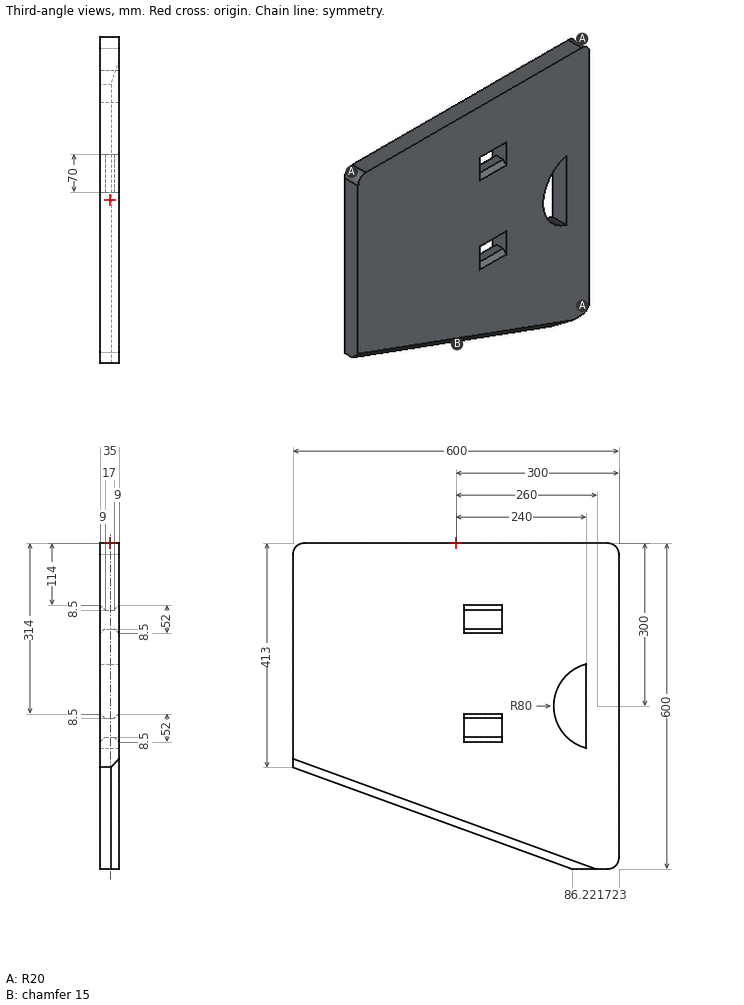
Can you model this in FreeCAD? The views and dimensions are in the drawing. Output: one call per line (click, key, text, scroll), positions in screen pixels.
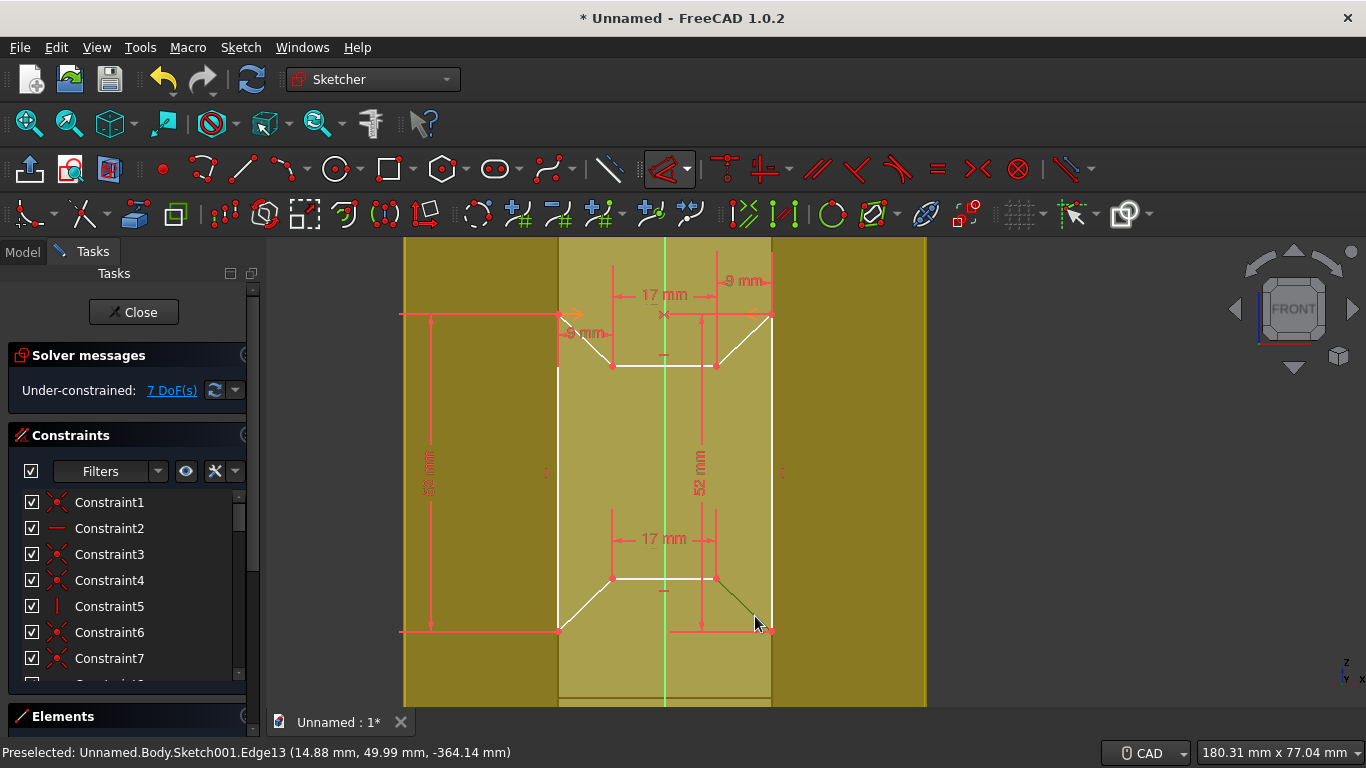
click(690, 170)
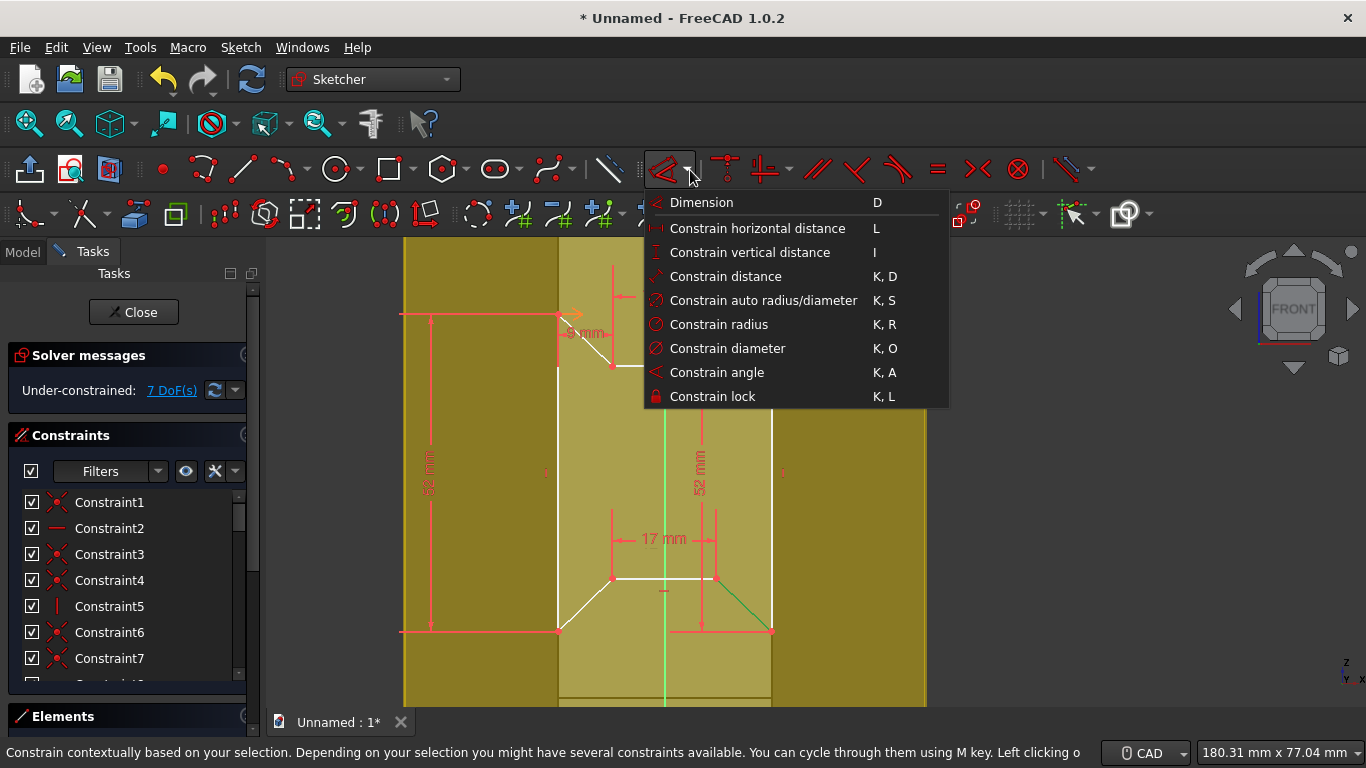
click(797, 228)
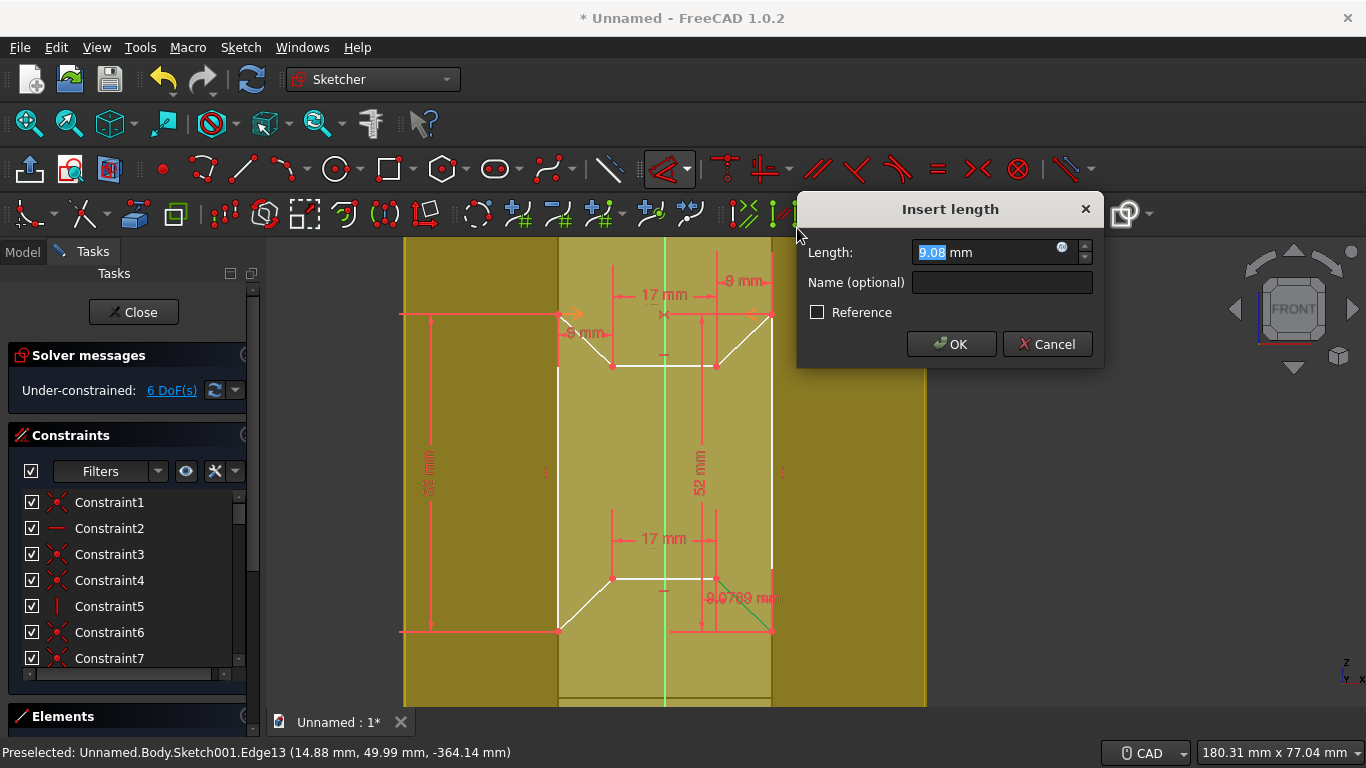
text(9)
key(Return)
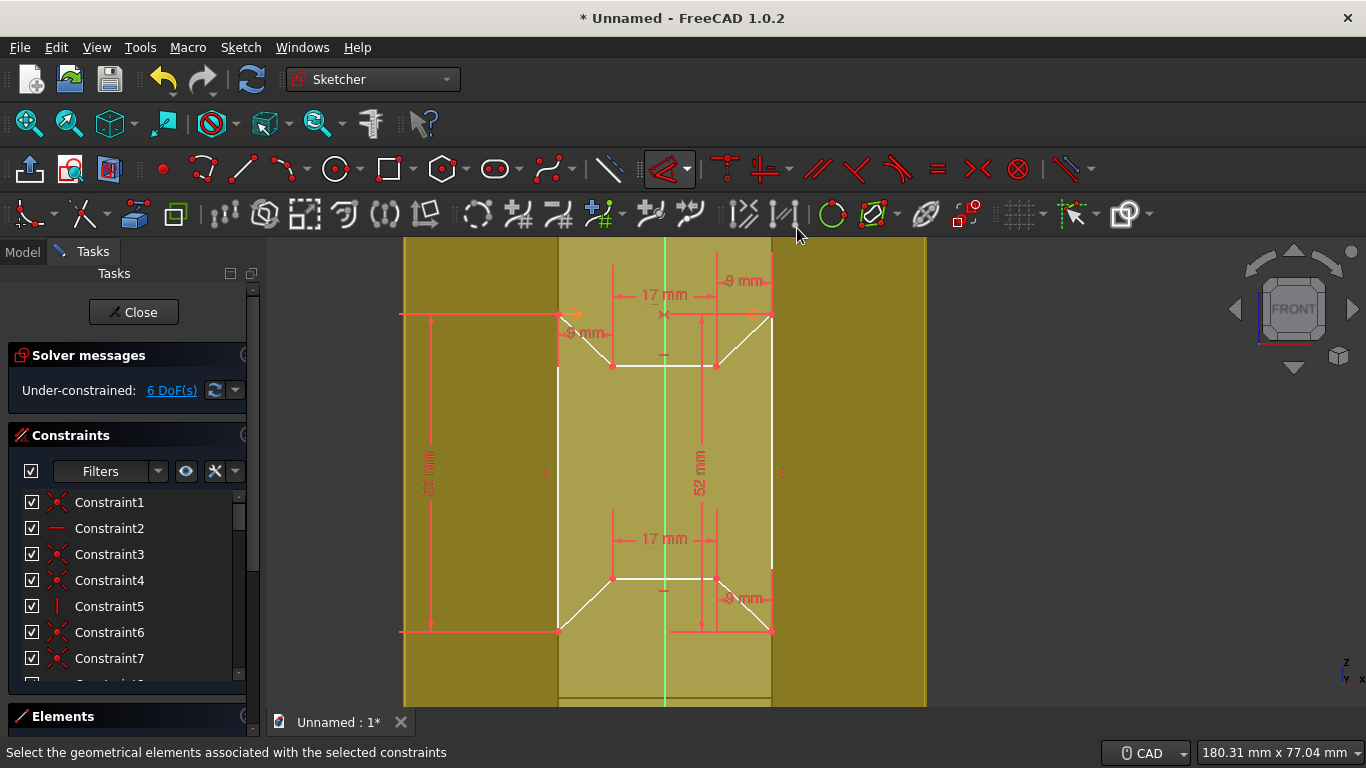
scroll(760, 622, down, 10)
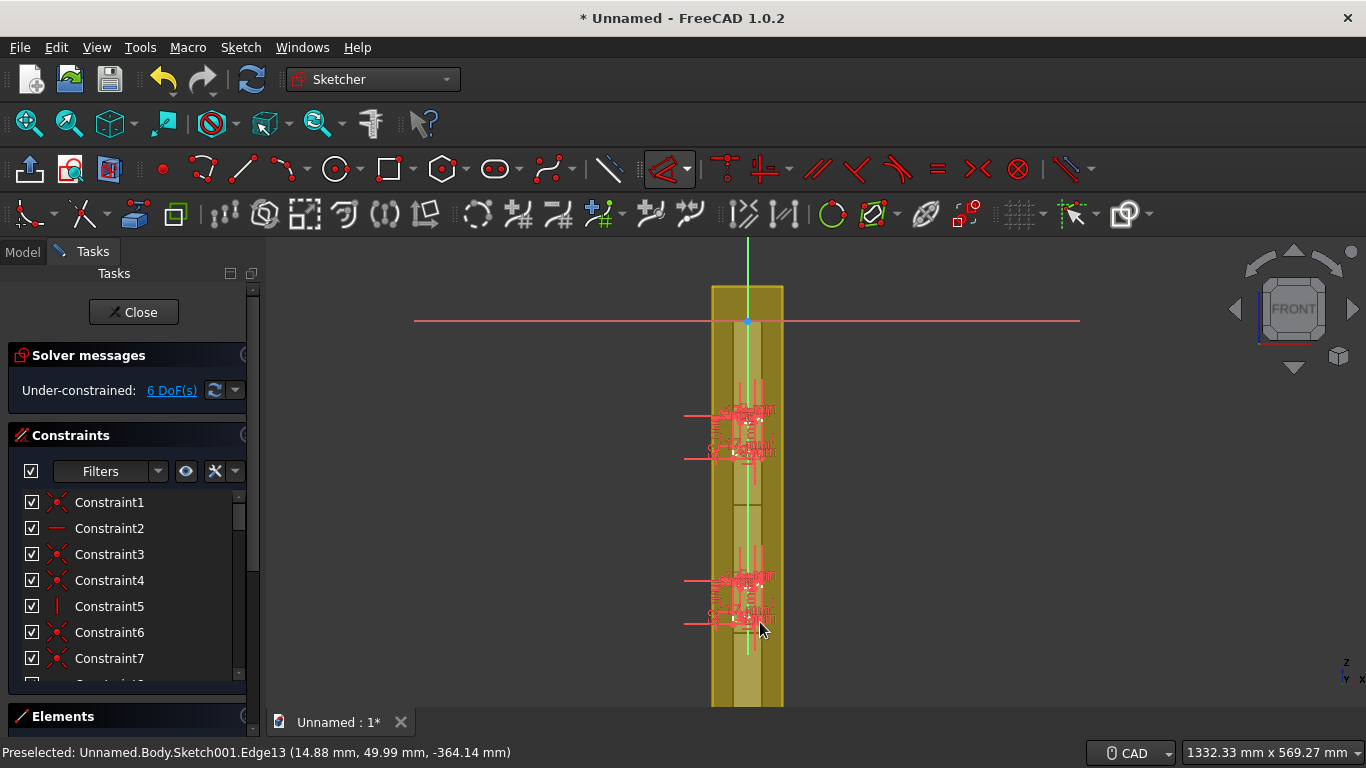
click(733, 416)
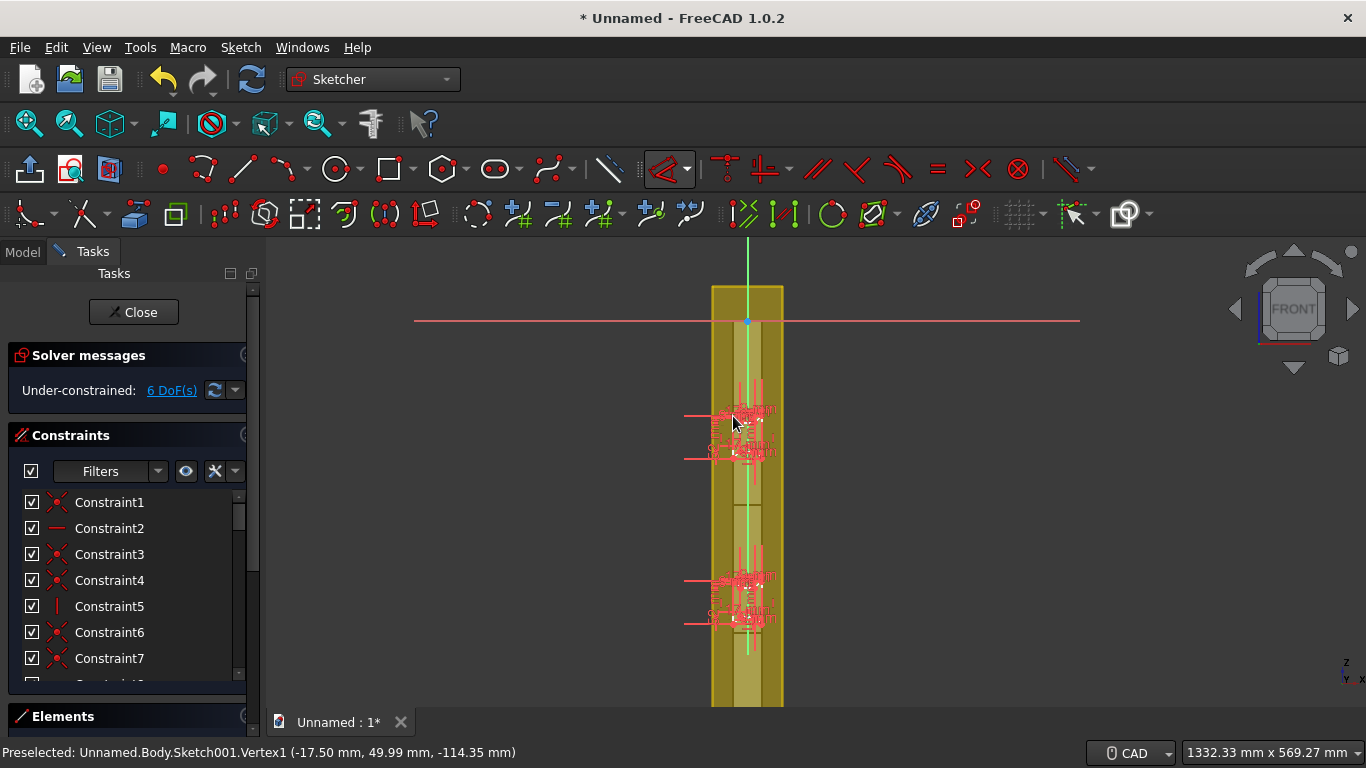
click(690, 170)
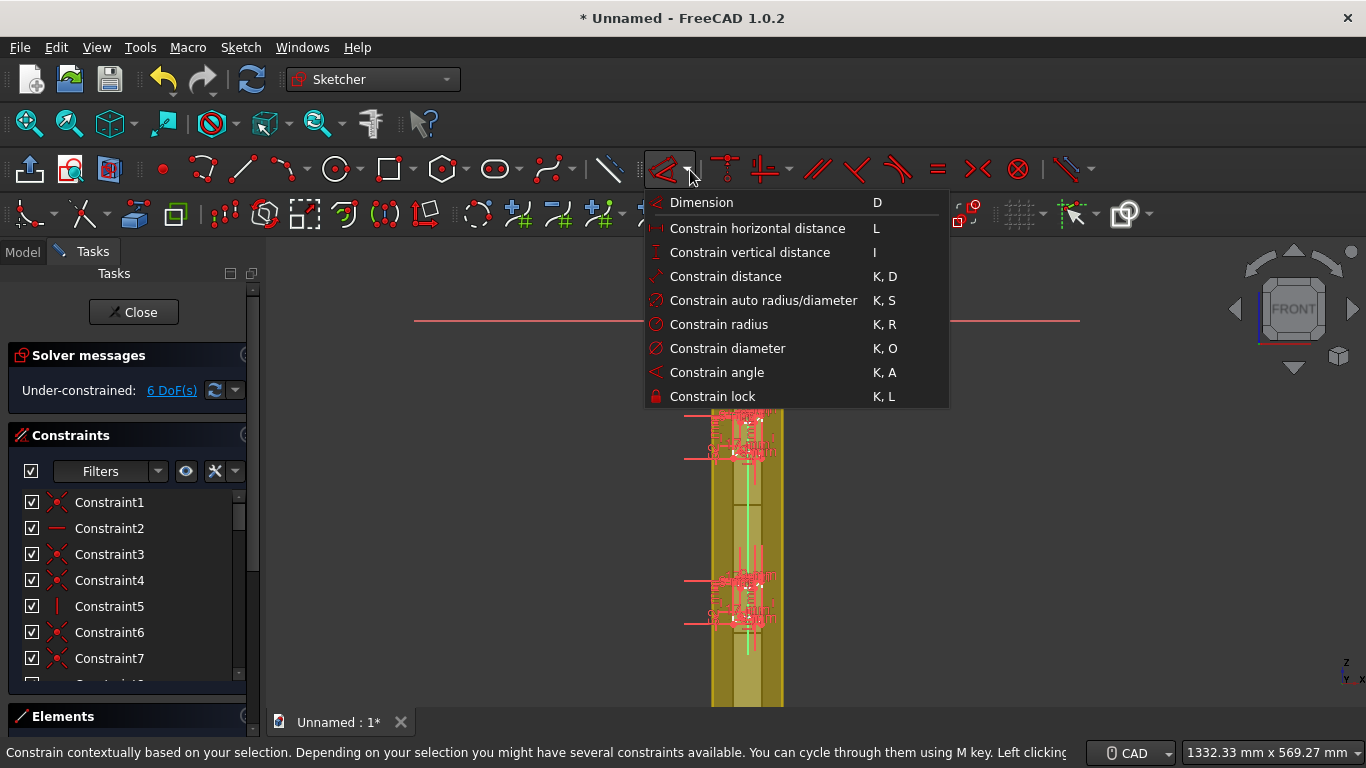
click(797, 252)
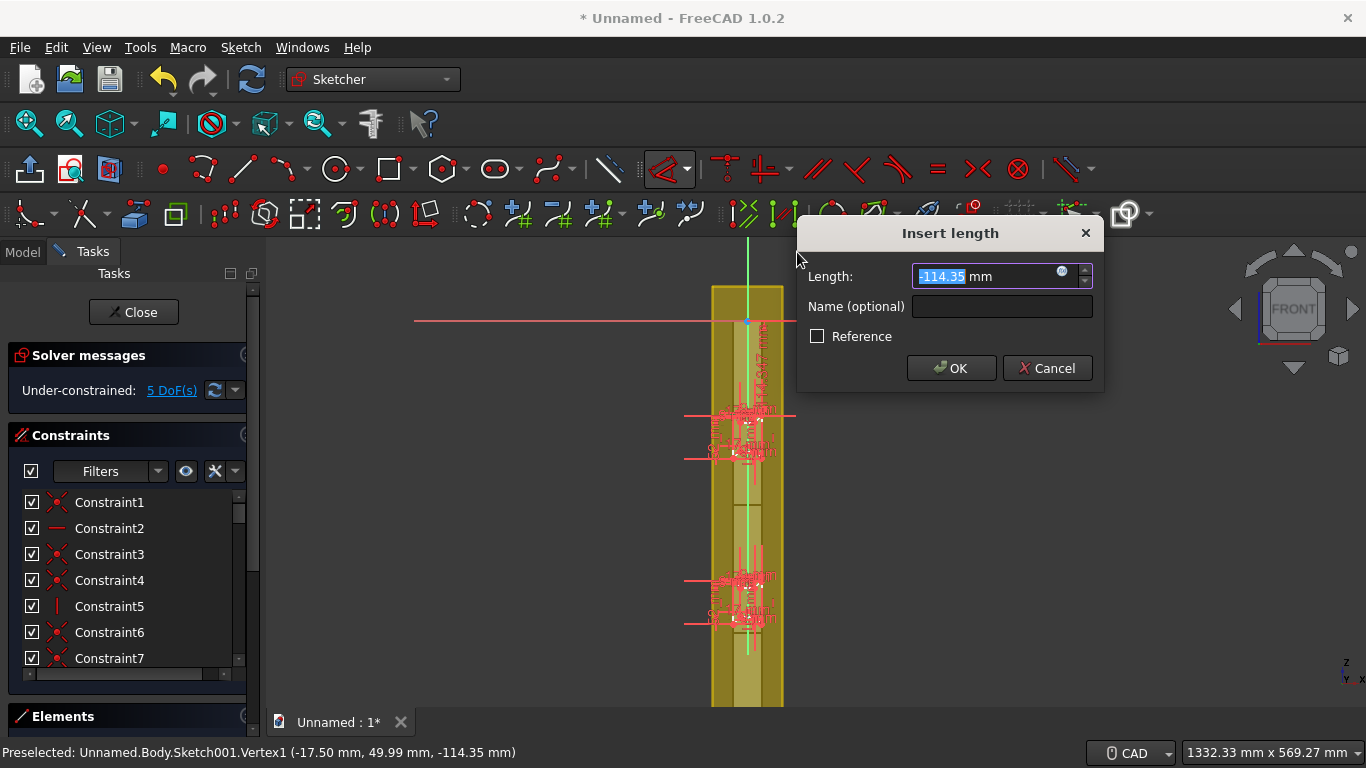
text(-114)
key(Return)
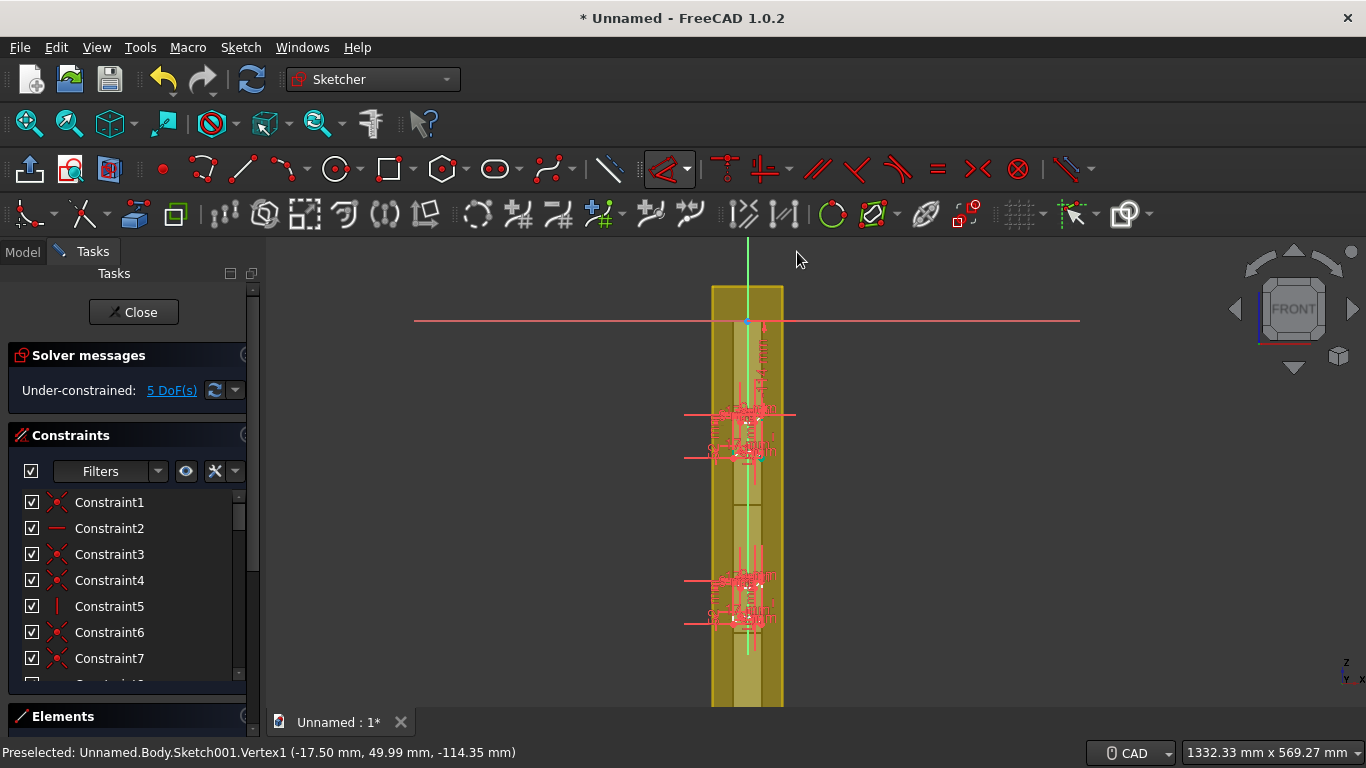
click(733, 581)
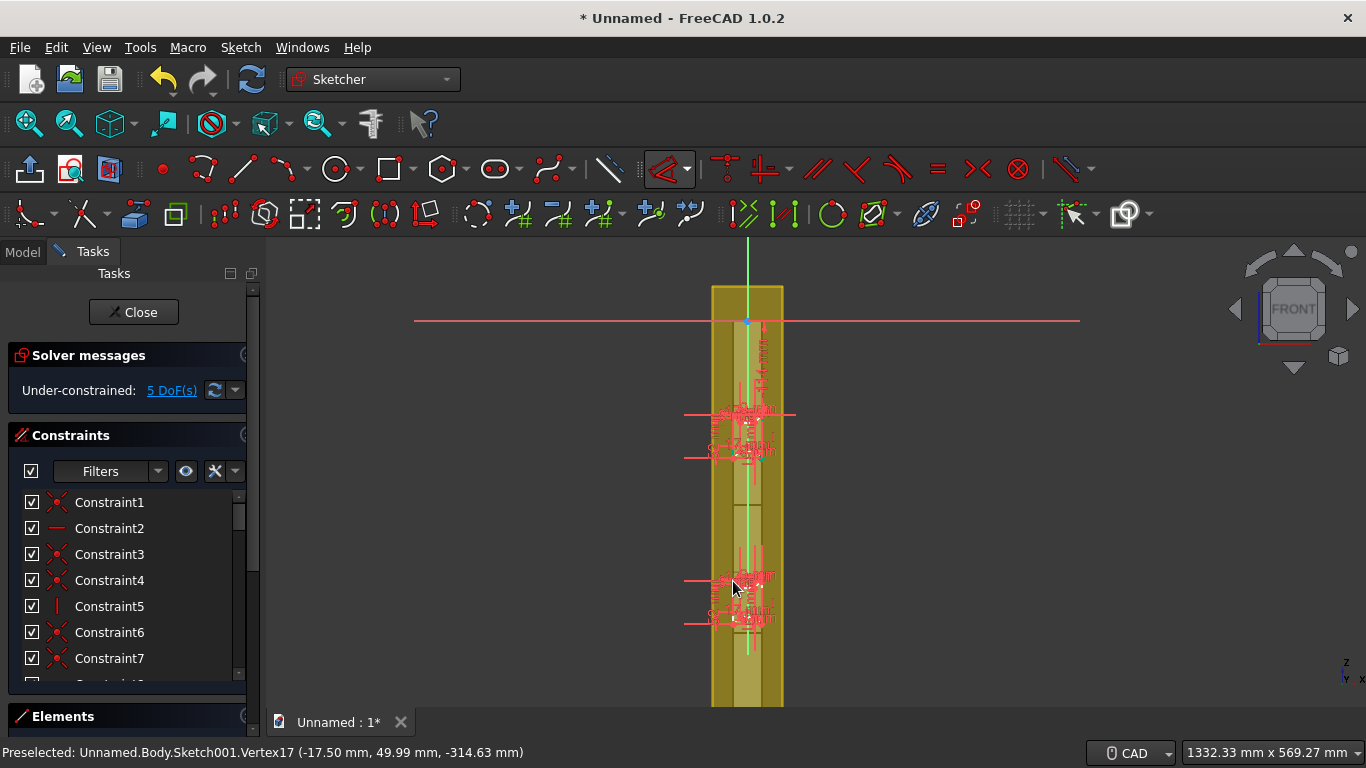
key(i)